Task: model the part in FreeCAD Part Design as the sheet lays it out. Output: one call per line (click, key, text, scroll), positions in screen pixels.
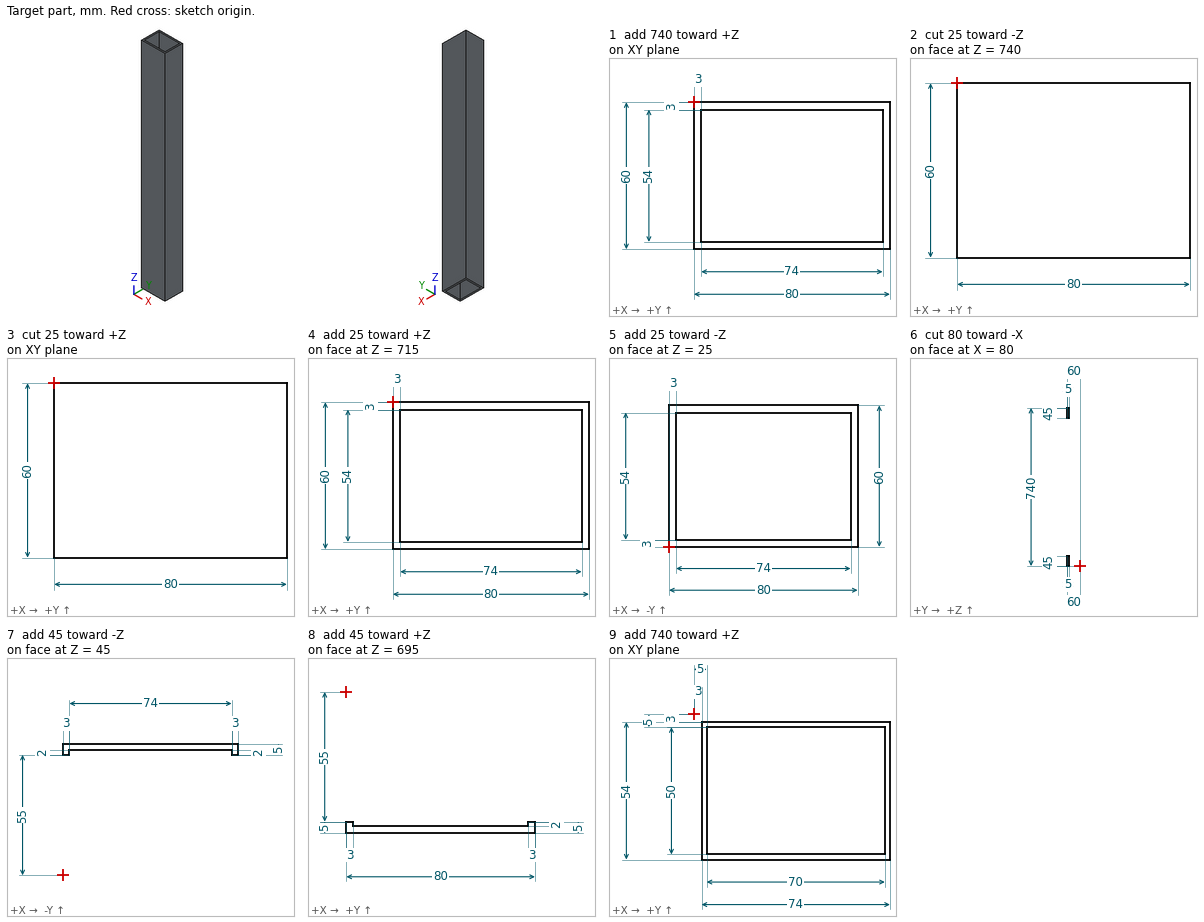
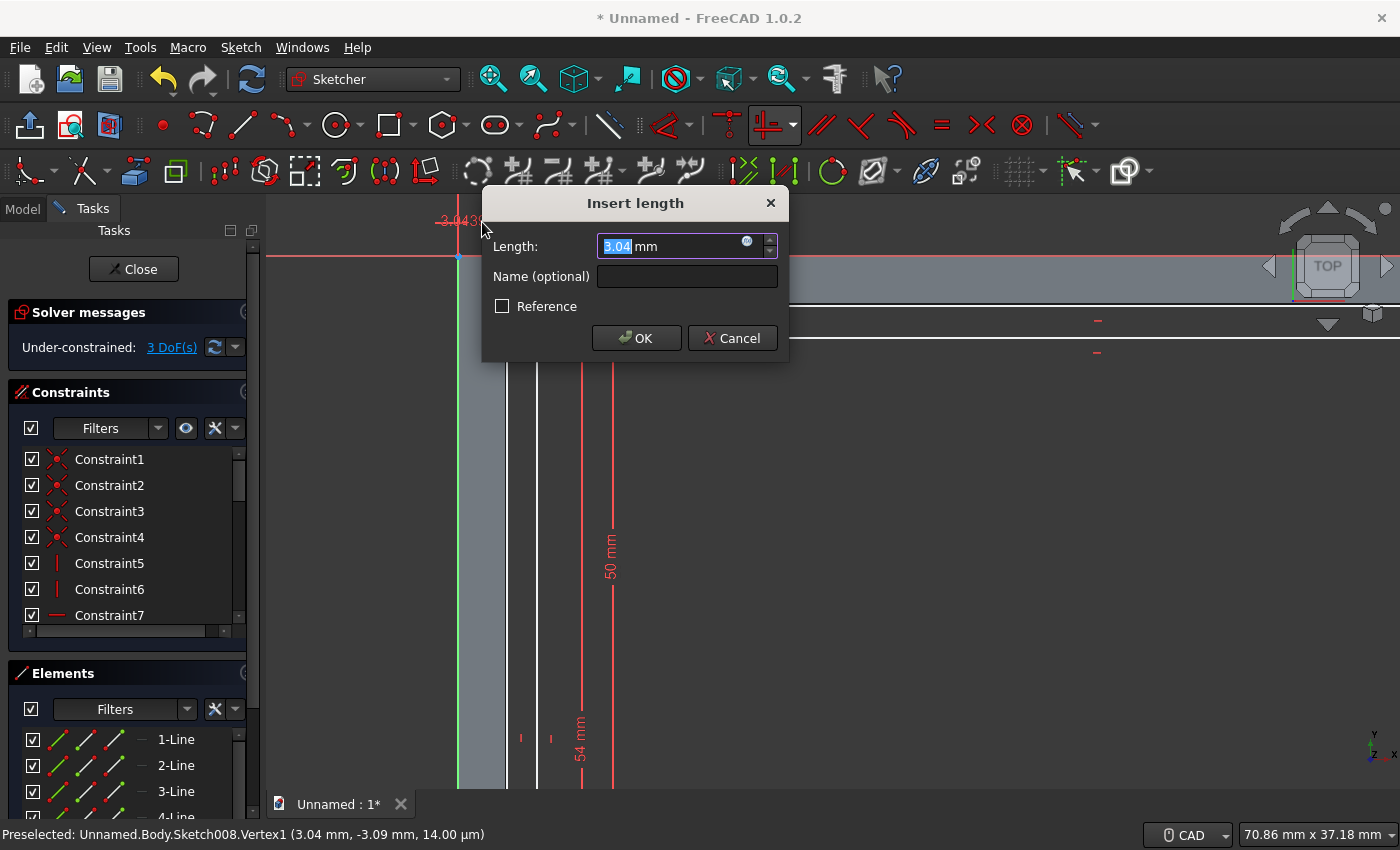
text(3)
key(Return)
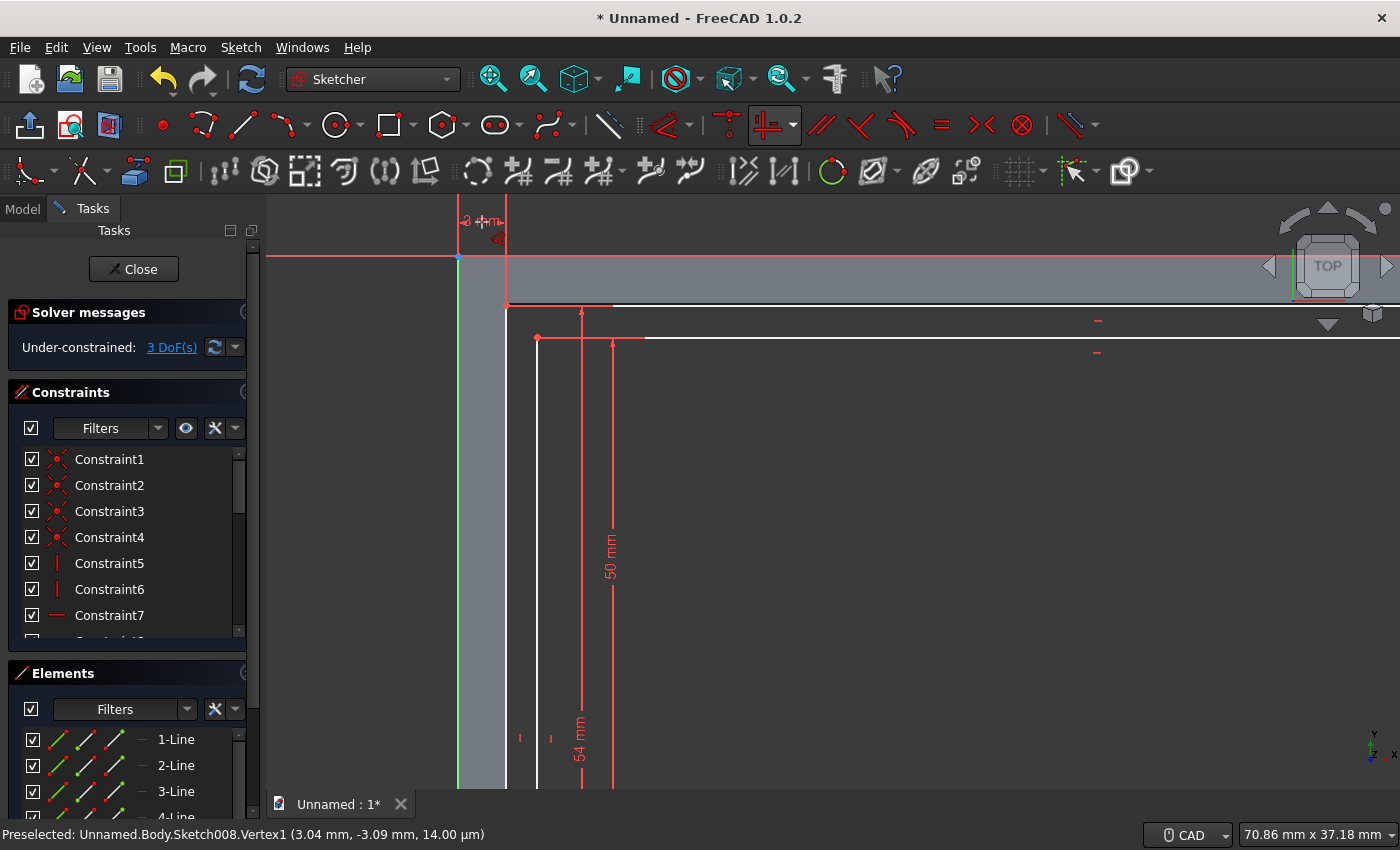
click(506, 306)
click(424, 281)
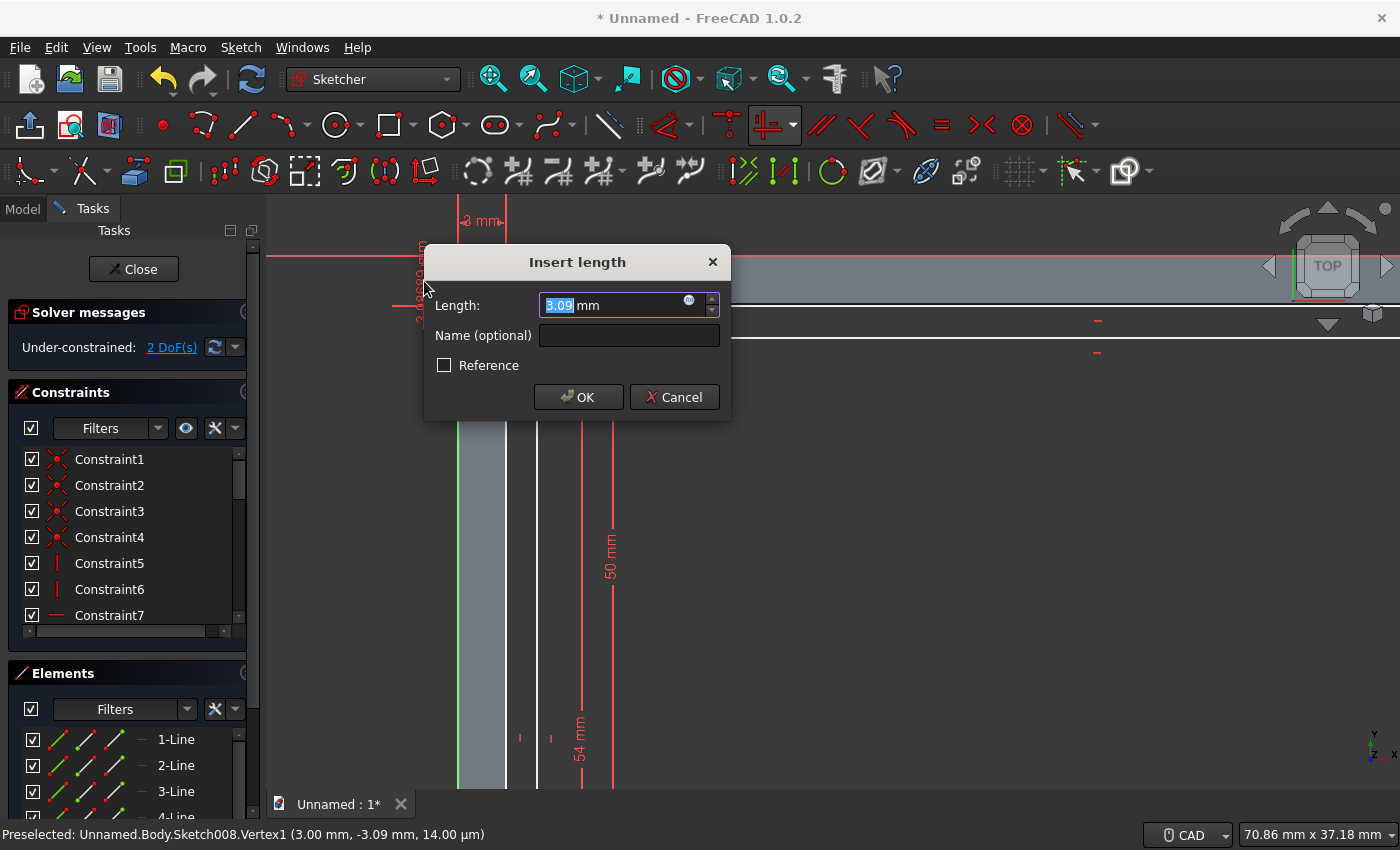
text(3)
key(Return)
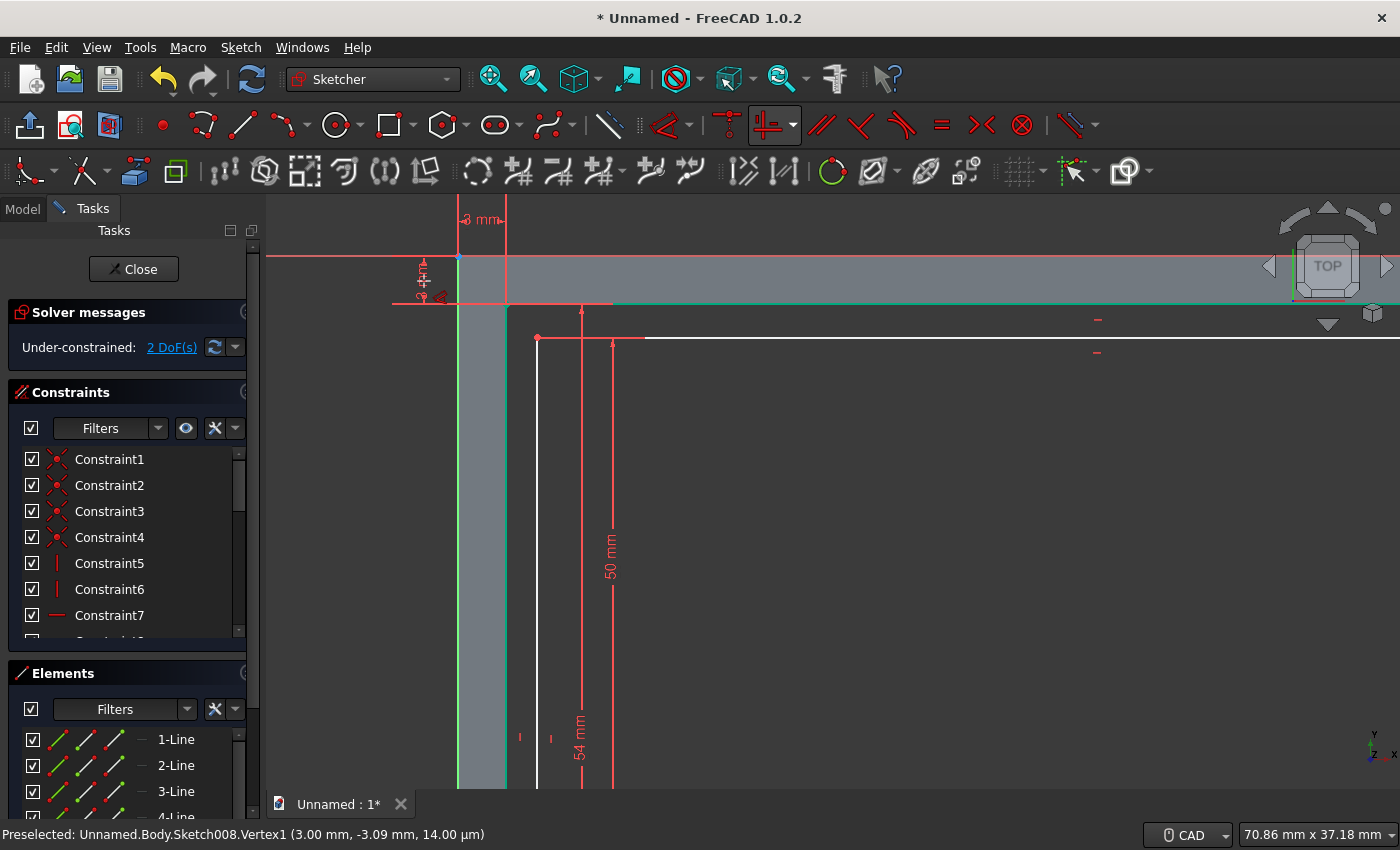
click(537, 338)
click(479, 372)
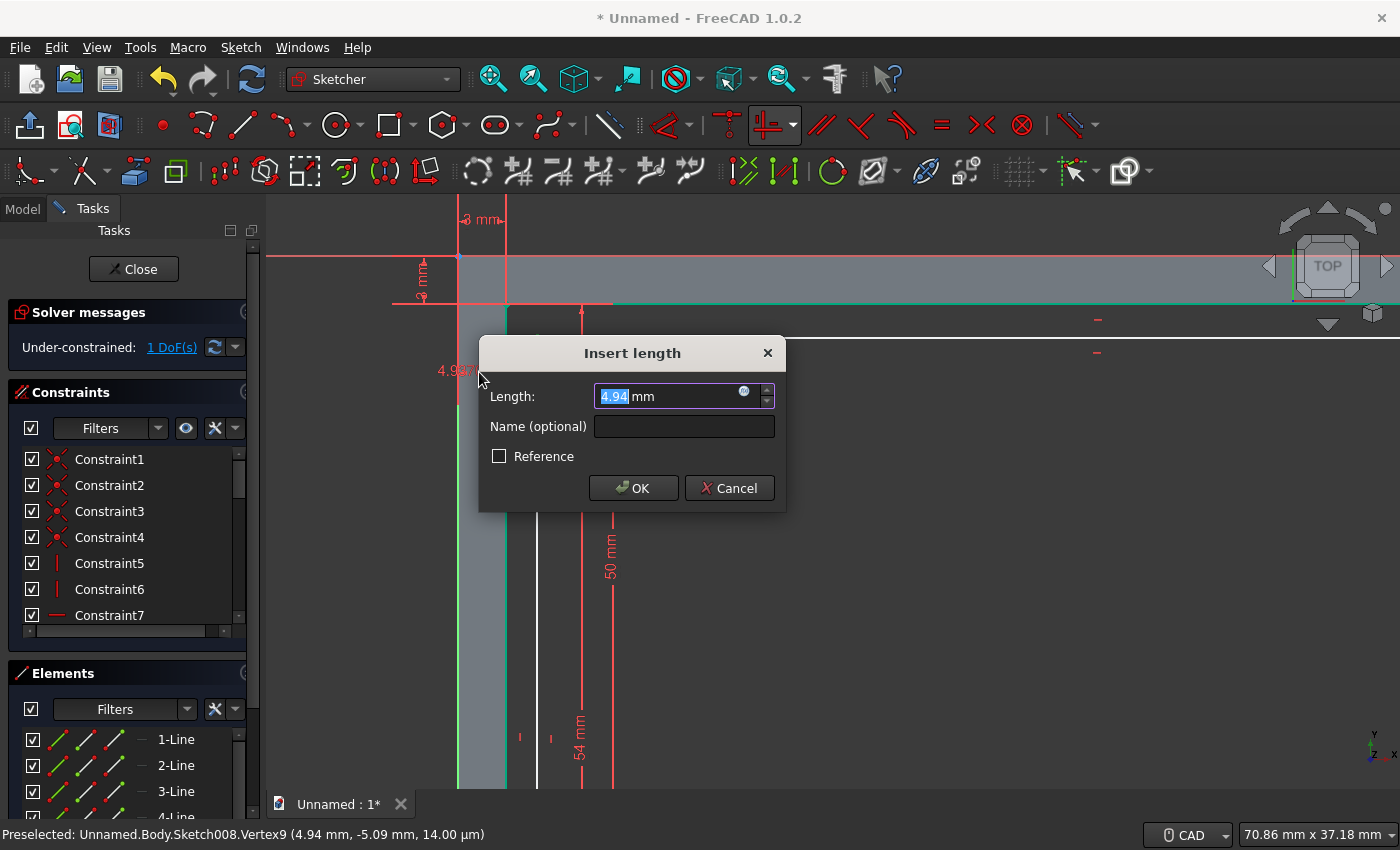
text(5)
key(Return)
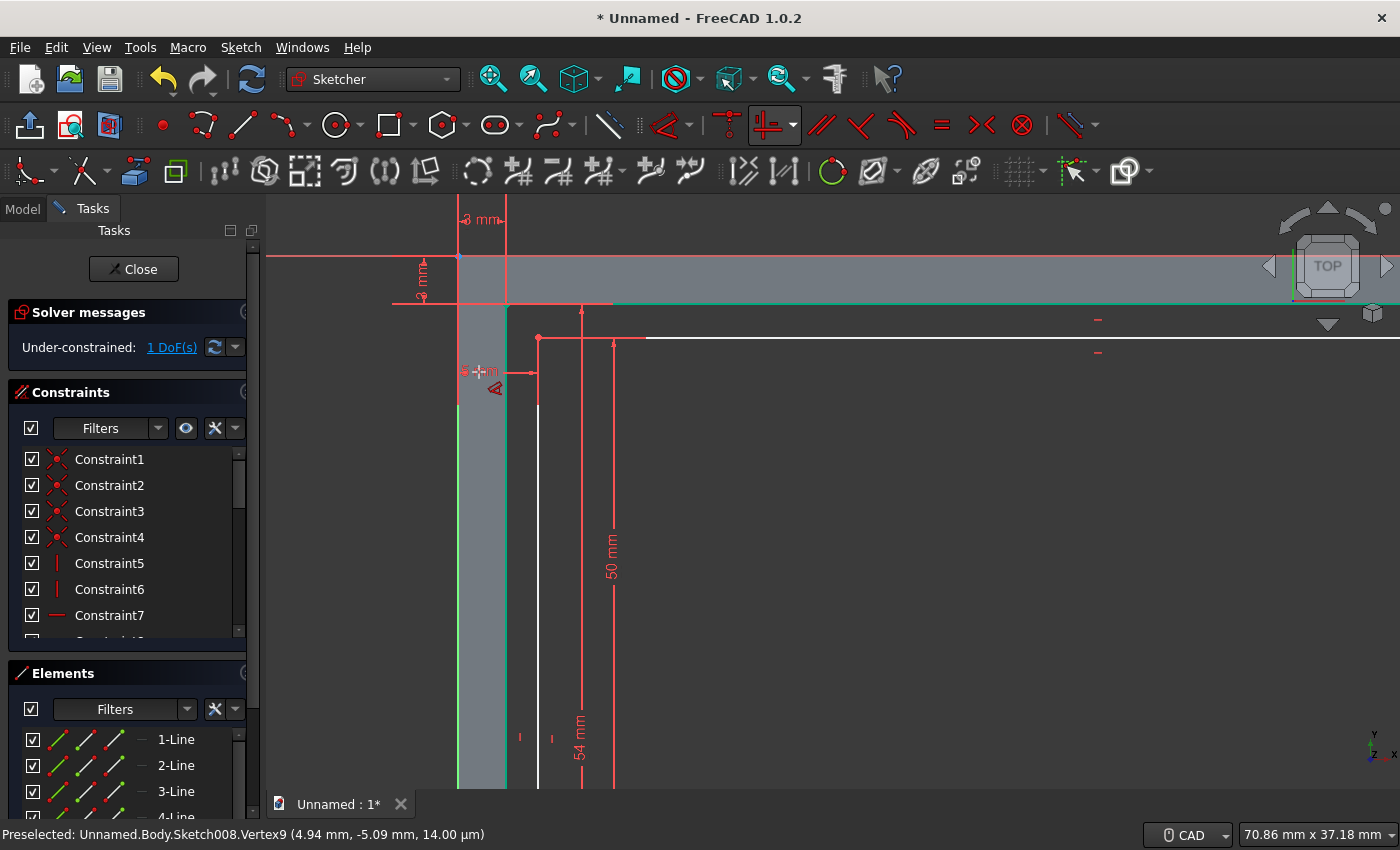
click(538, 338)
click(424, 316)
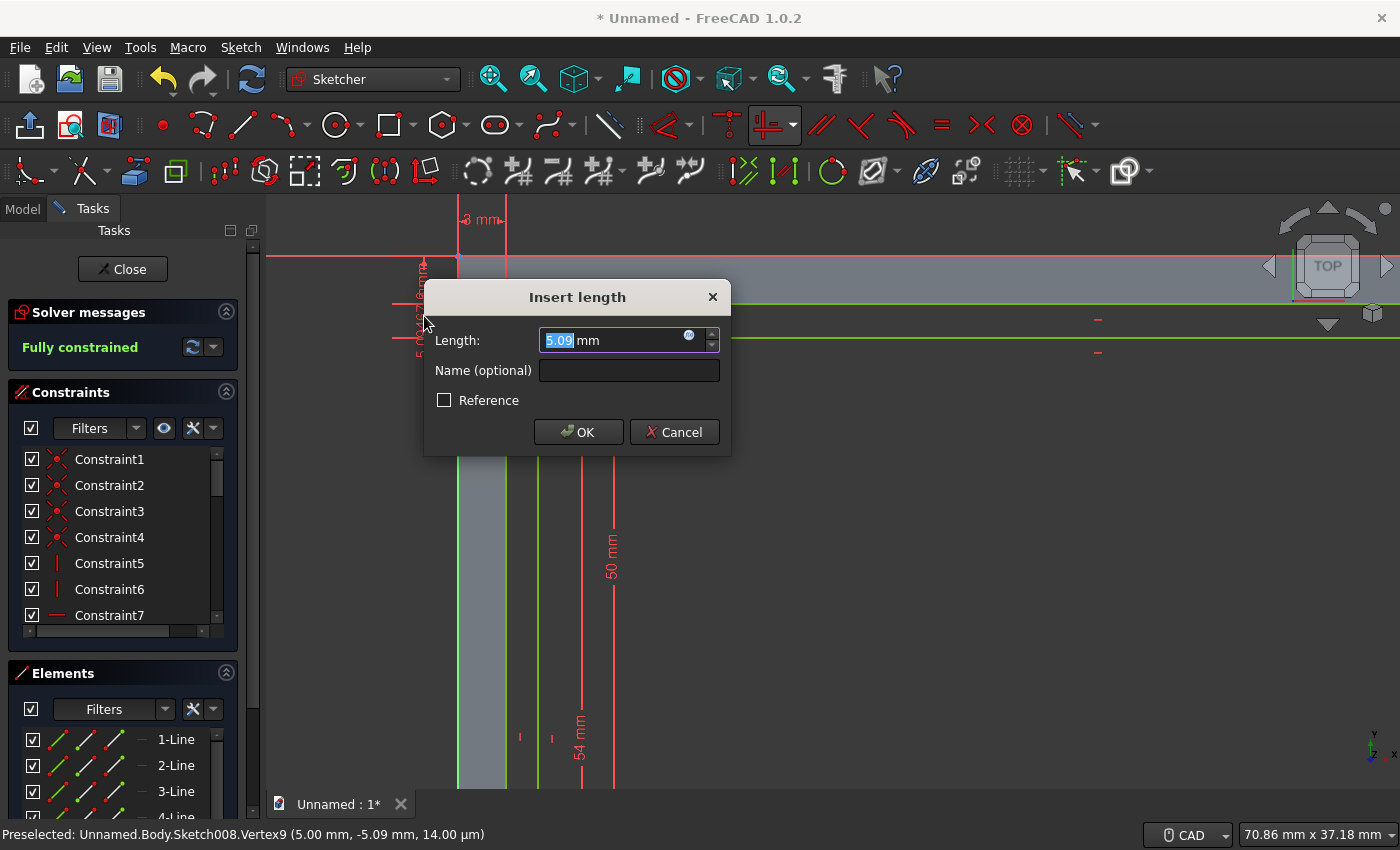
text(5)
key(Return)
key(Escape)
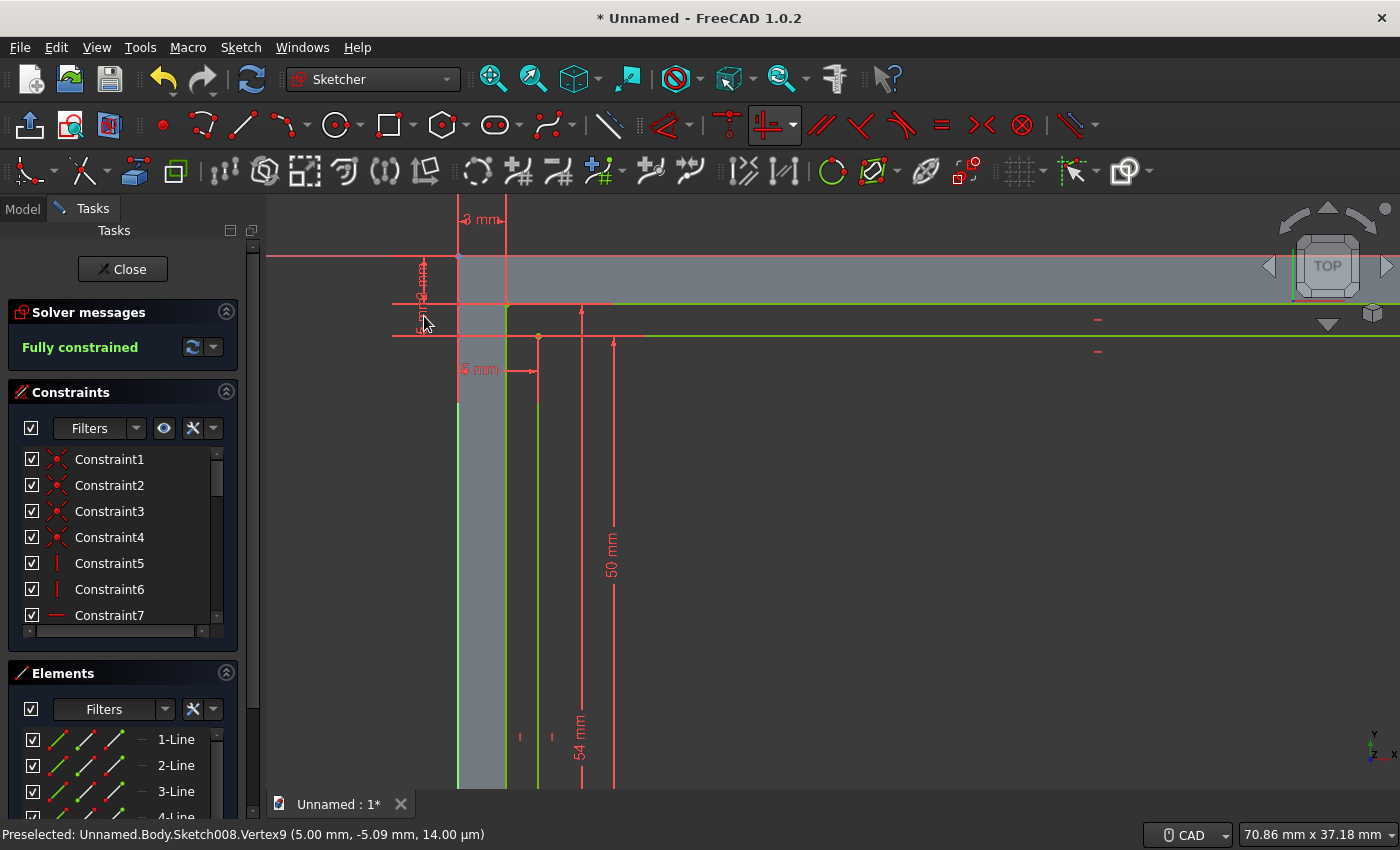
click(123, 269)